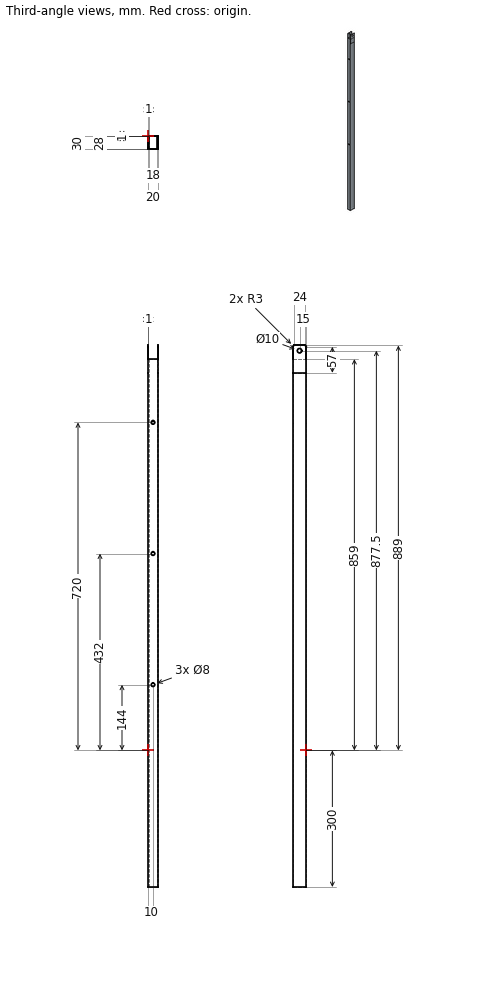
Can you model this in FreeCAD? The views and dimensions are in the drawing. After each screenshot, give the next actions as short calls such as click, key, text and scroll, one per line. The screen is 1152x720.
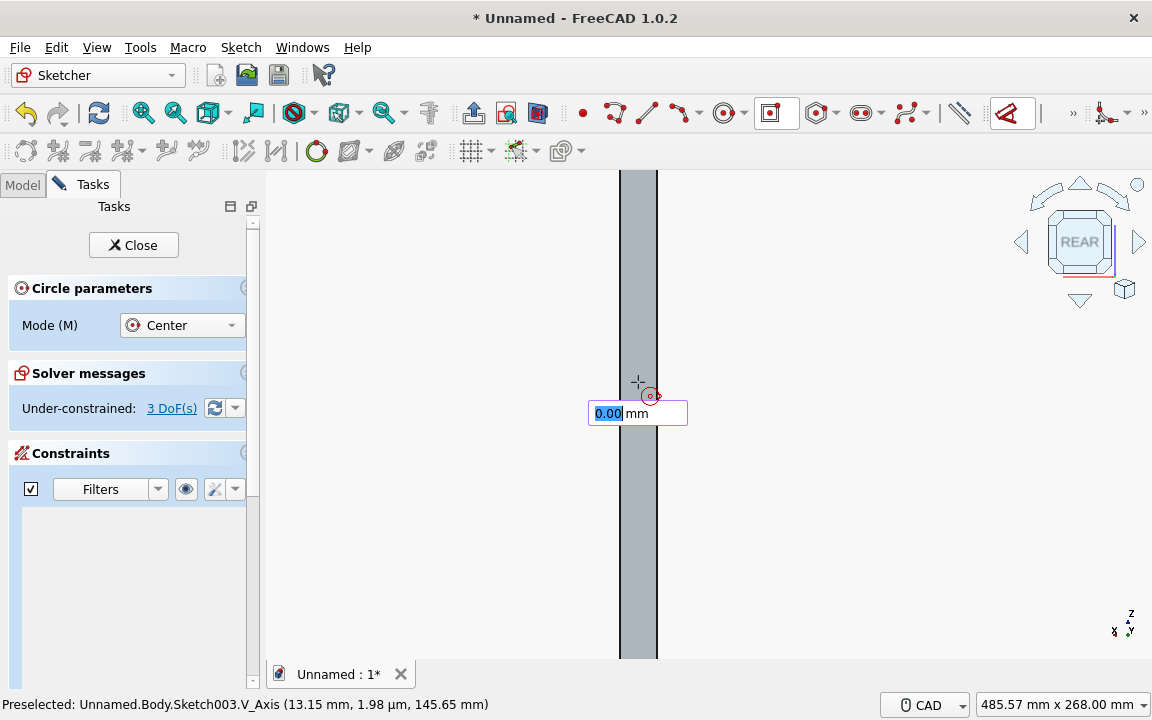
scroll(633, 377, up, 4)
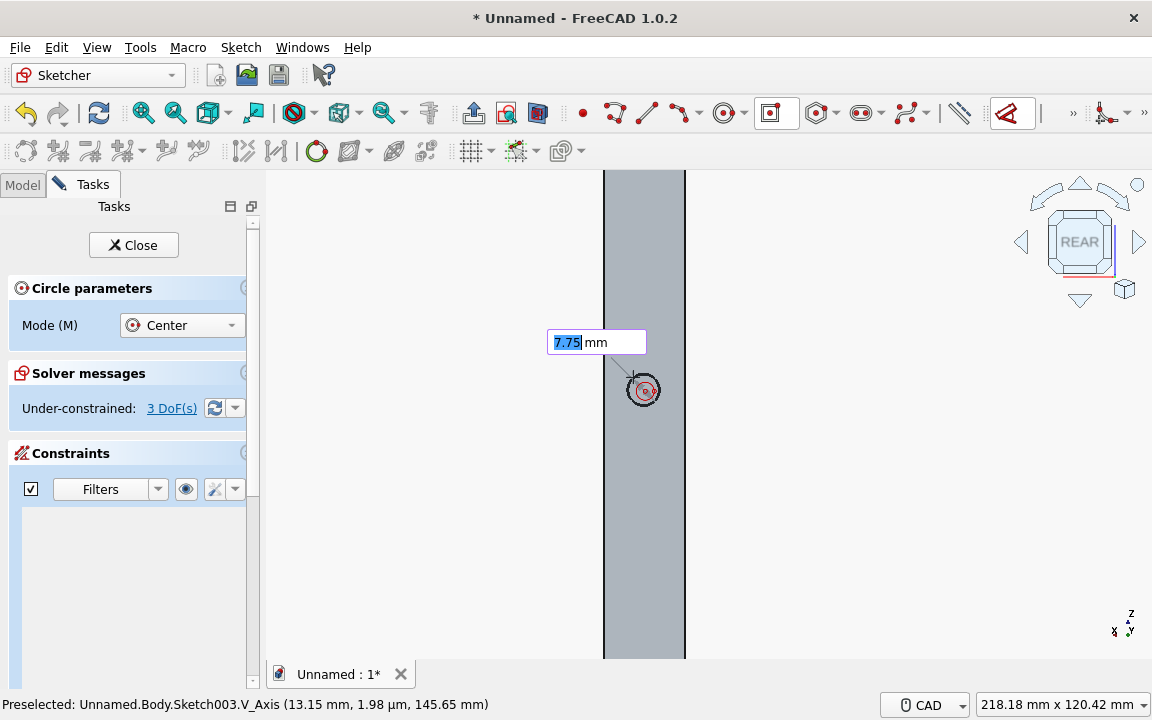
click(633, 376)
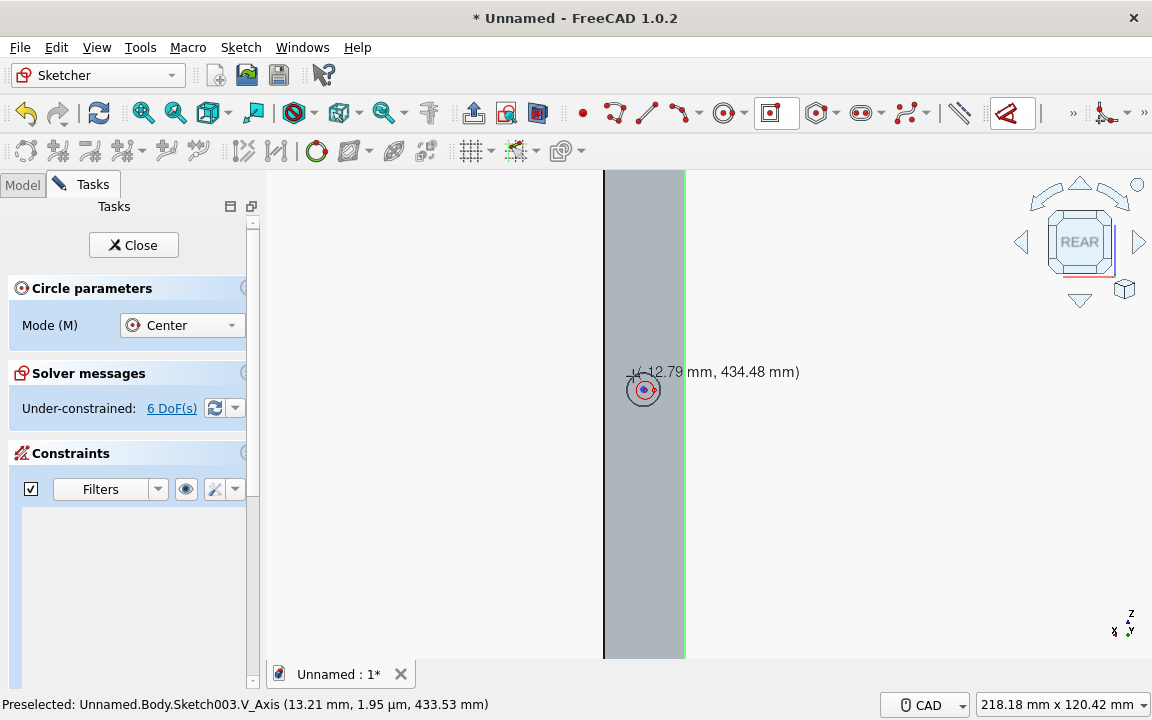
scroll(639, 382, down, 11)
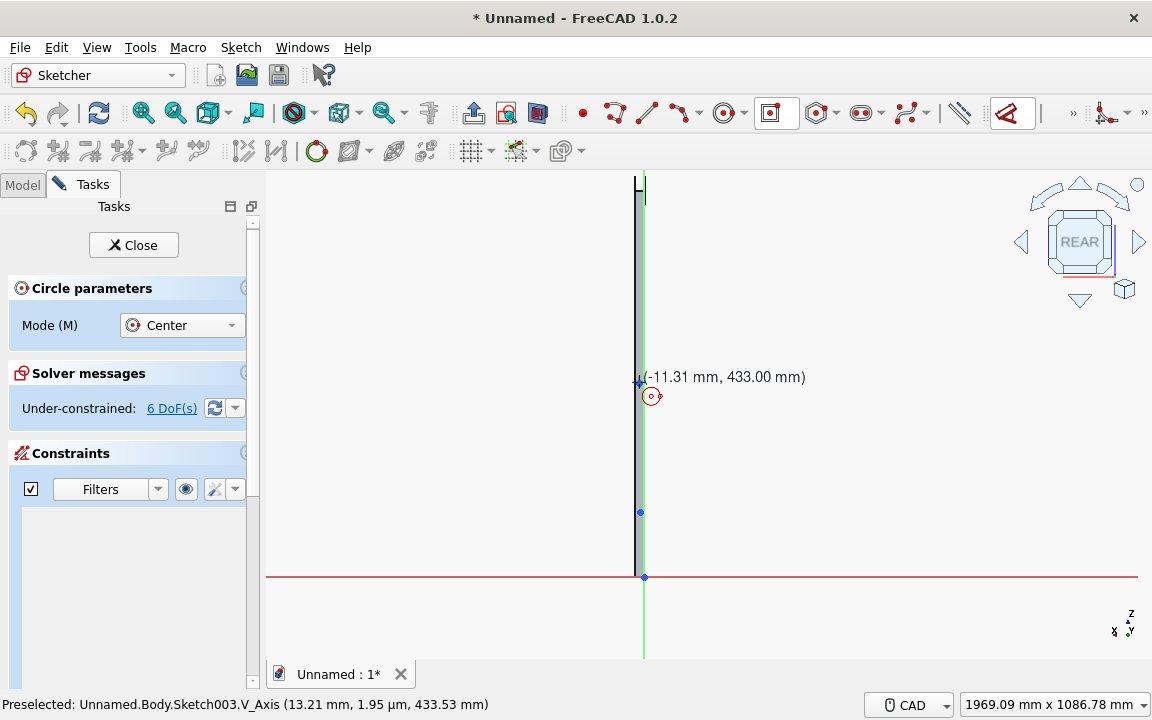
scroll(640, 253, up, 13)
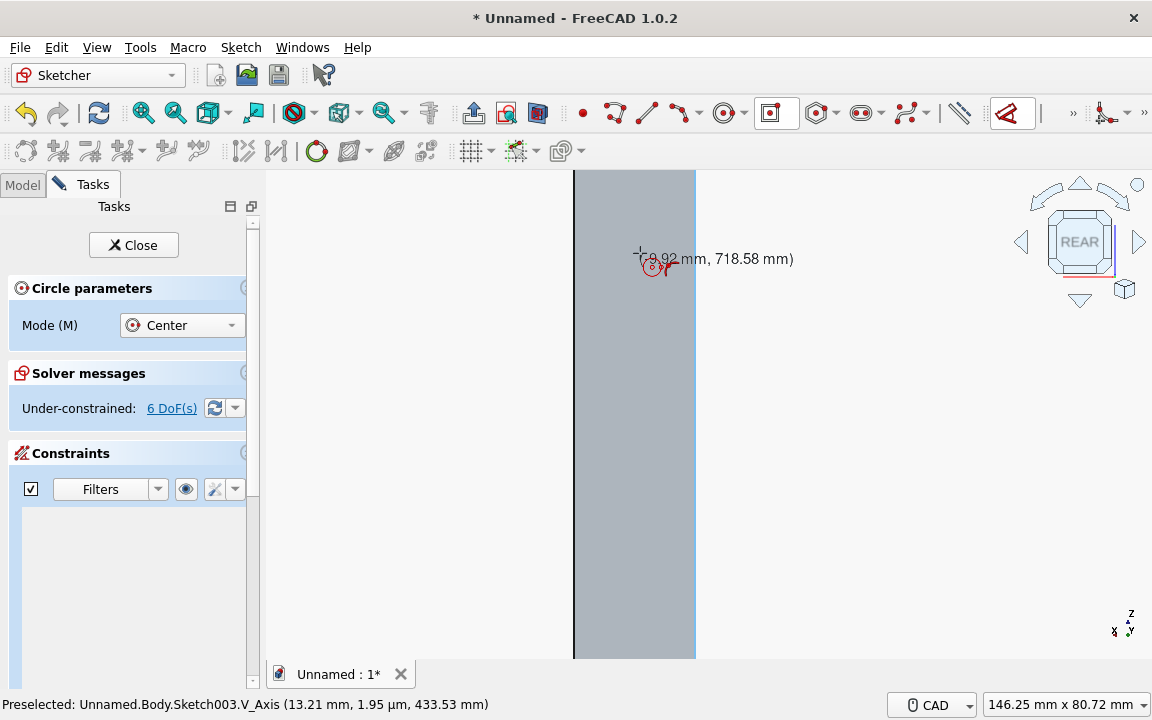
scroll(640, 253, down, 13)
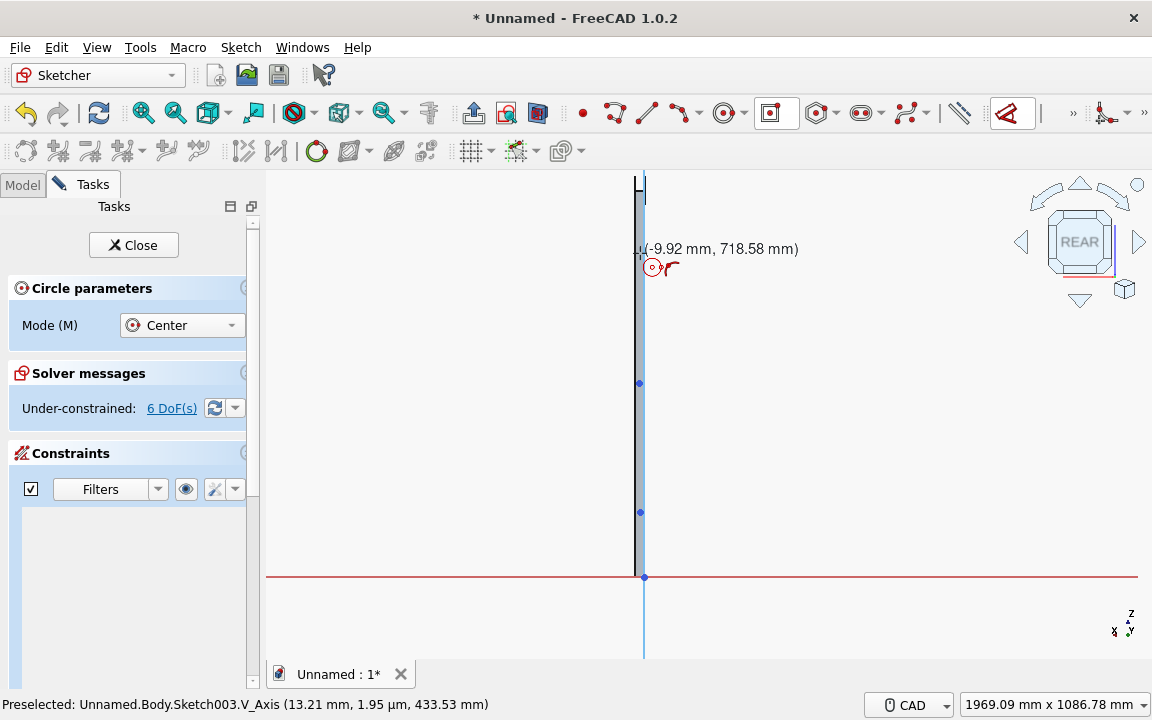
scroll(640, 253, up, 7)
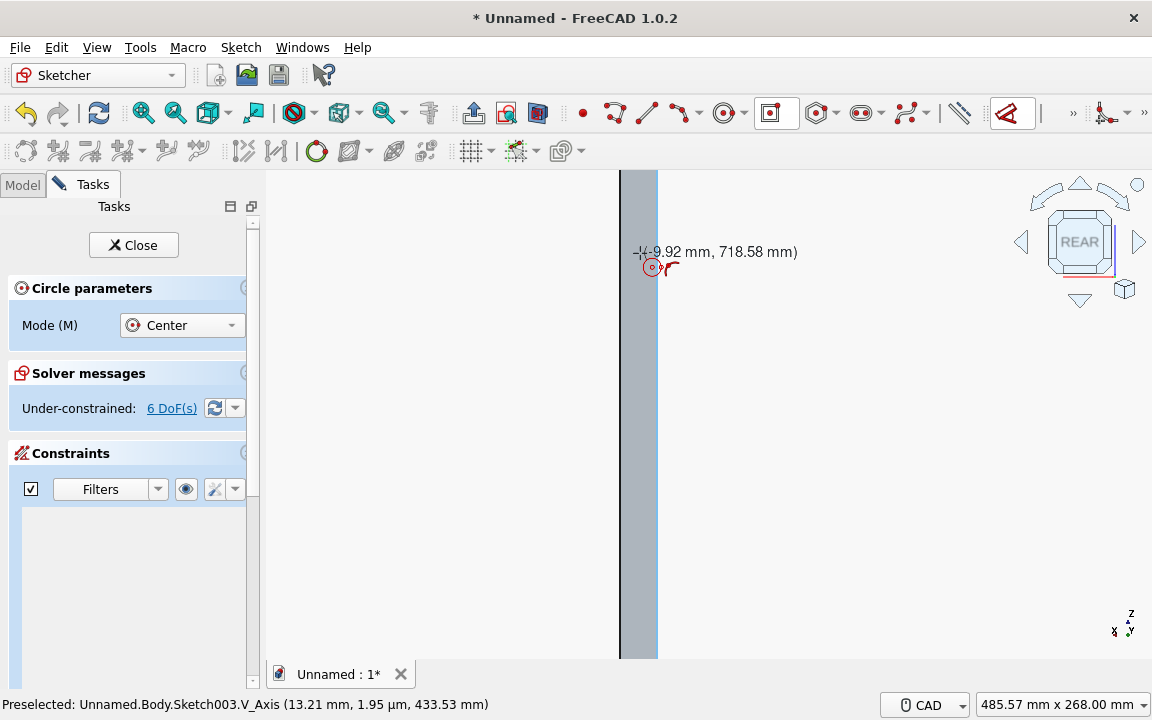
click(639, 254)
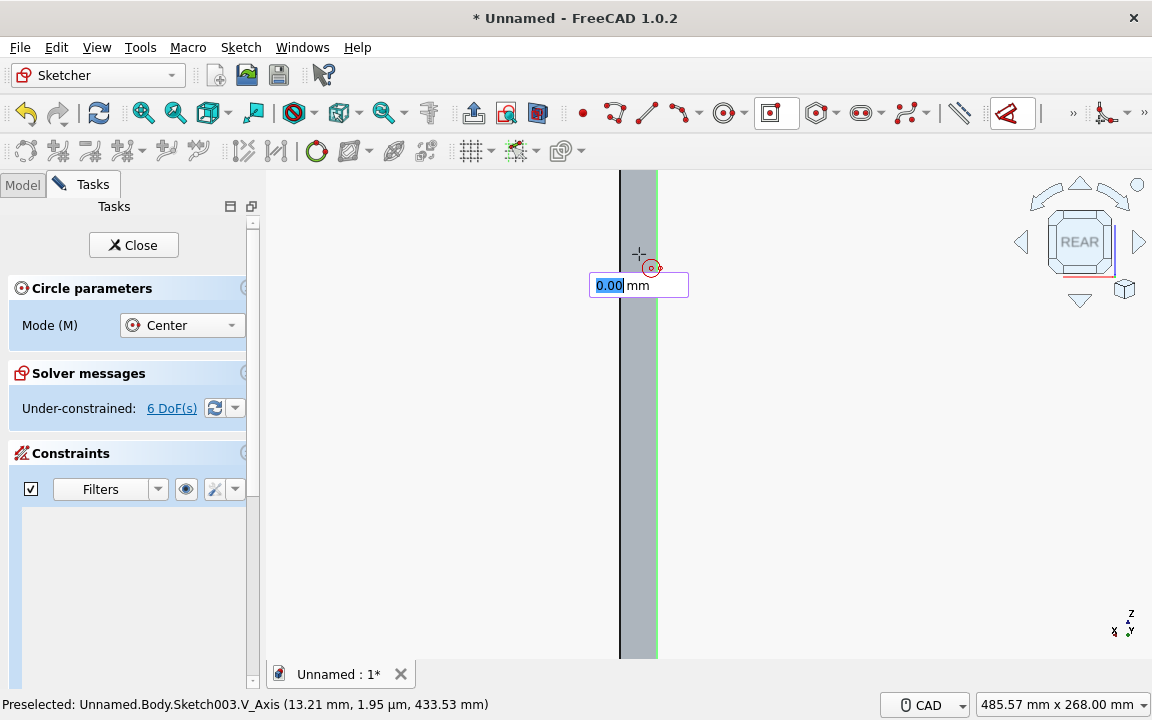
scroll(633, 249, up, 4)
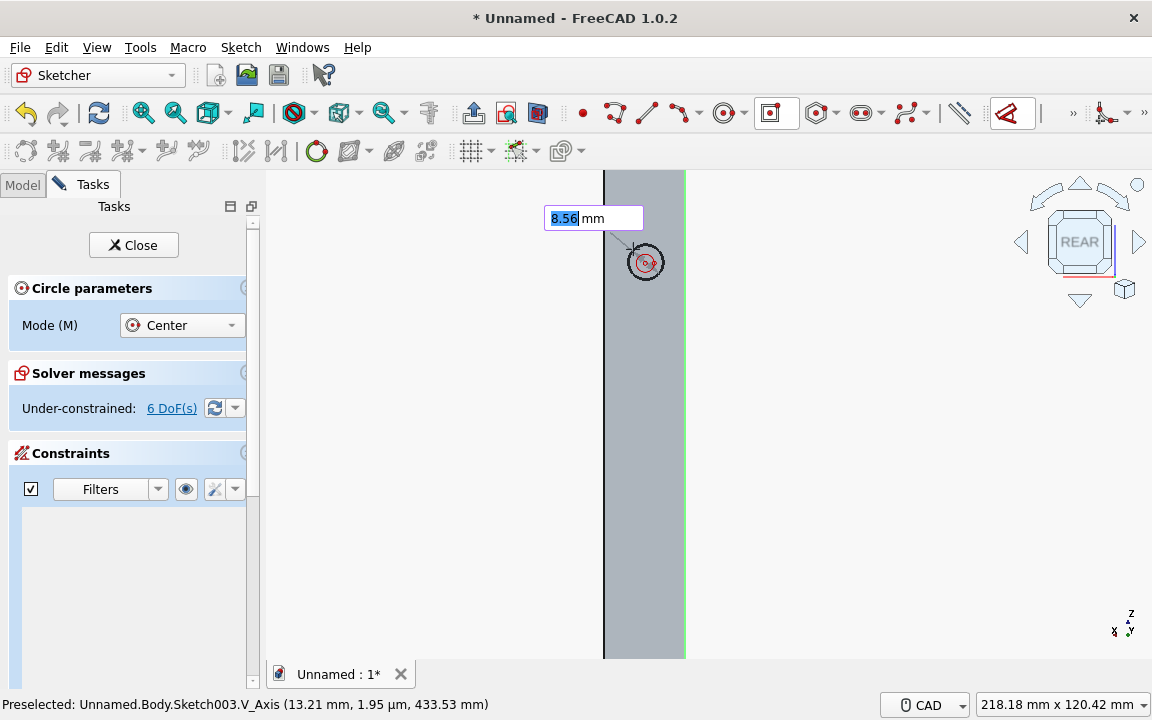
click(633, 248)
key(Escape)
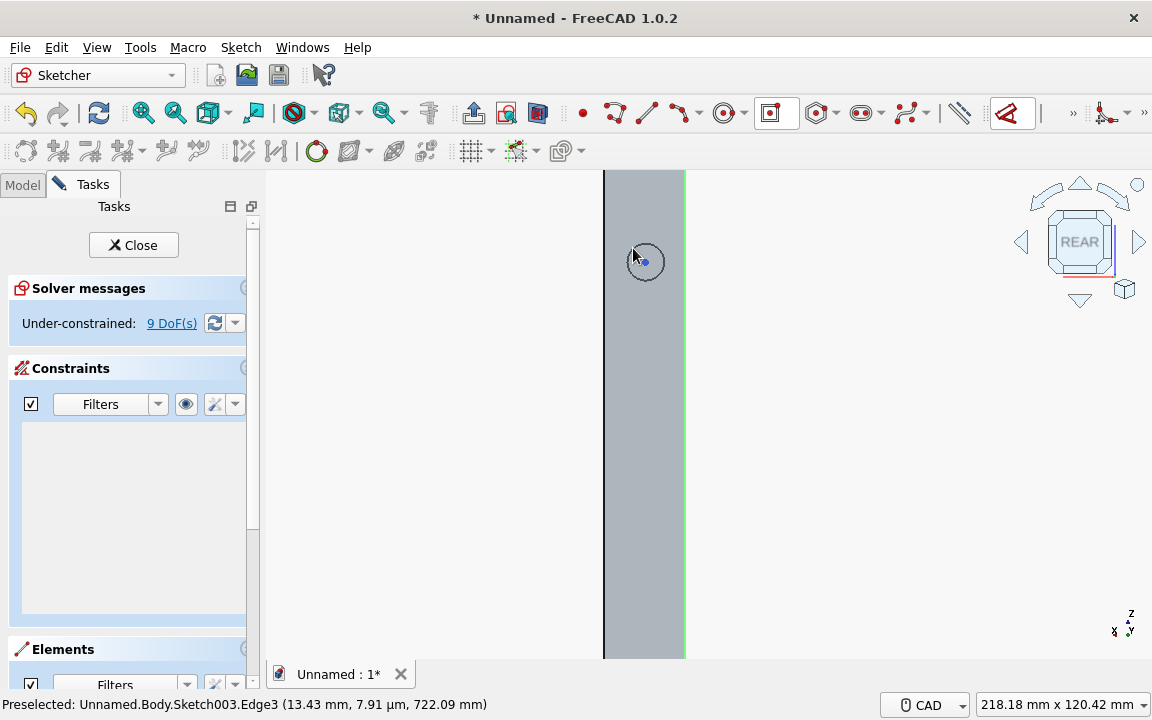
scroll(638, 253, down, 11)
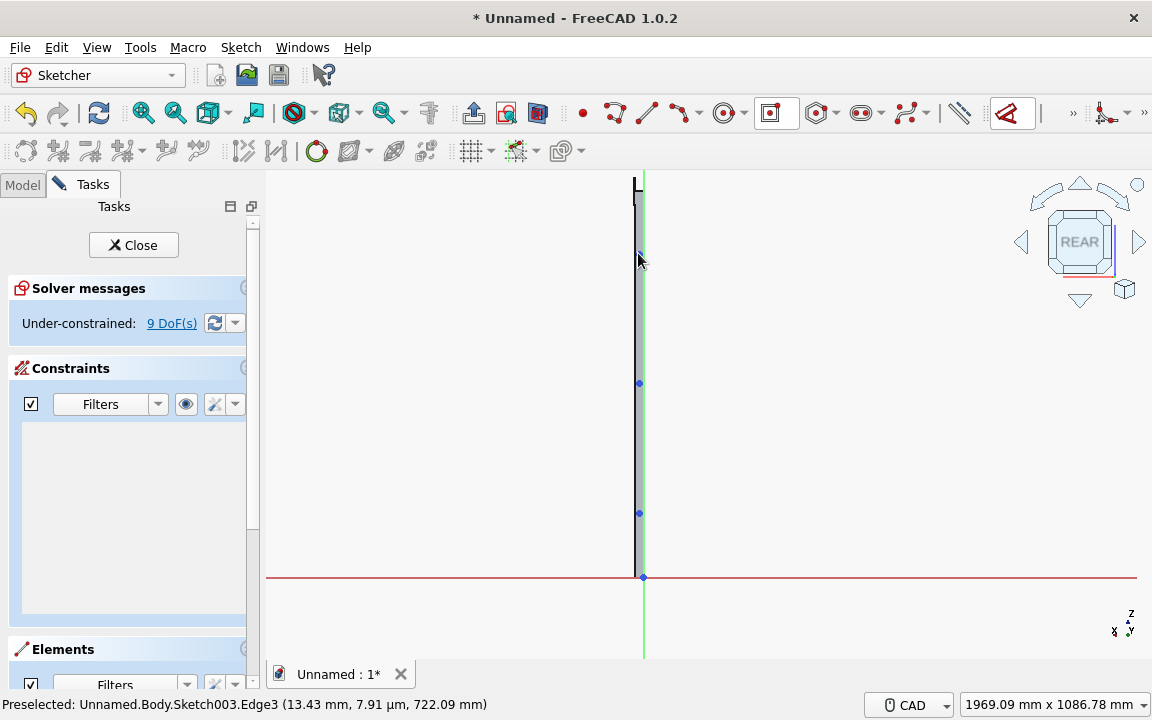
scroll(641, 512, up, 10)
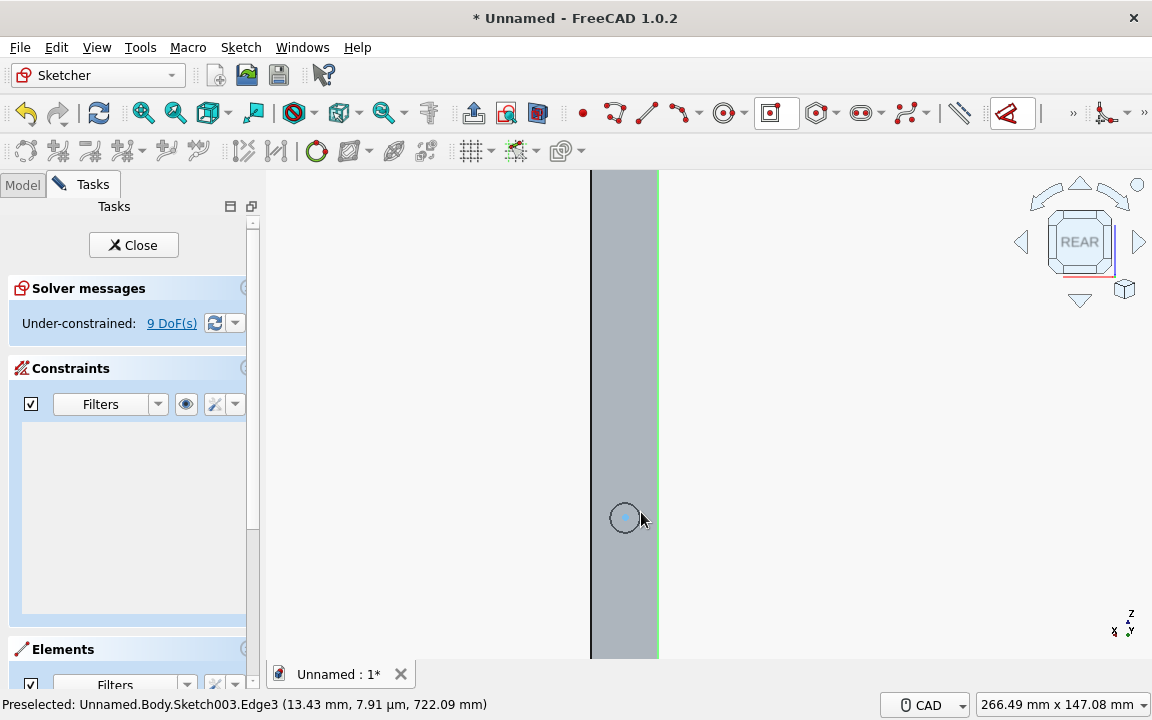
click(635, 508)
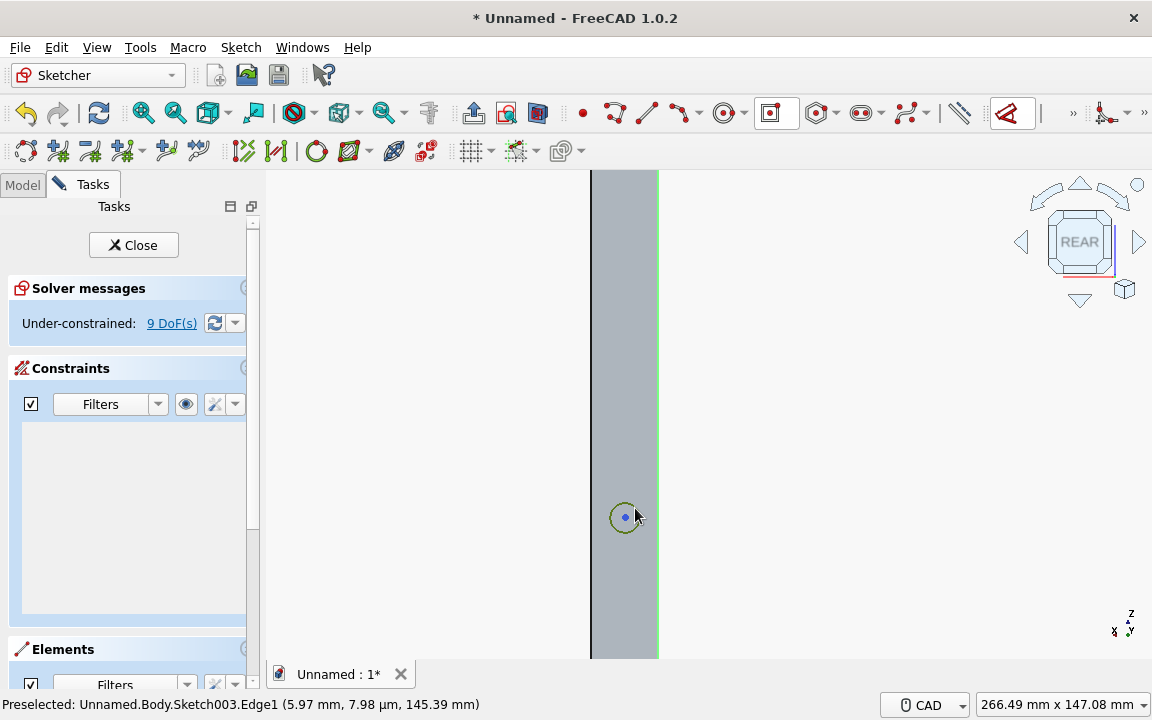
scroll(641, 512, down, 10)